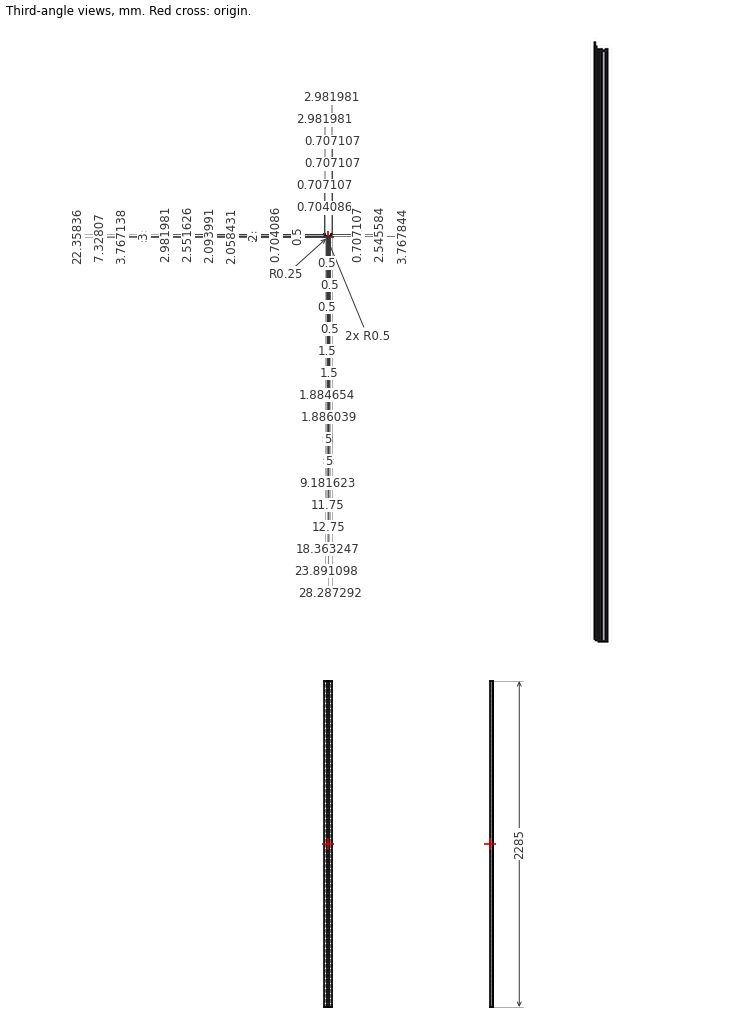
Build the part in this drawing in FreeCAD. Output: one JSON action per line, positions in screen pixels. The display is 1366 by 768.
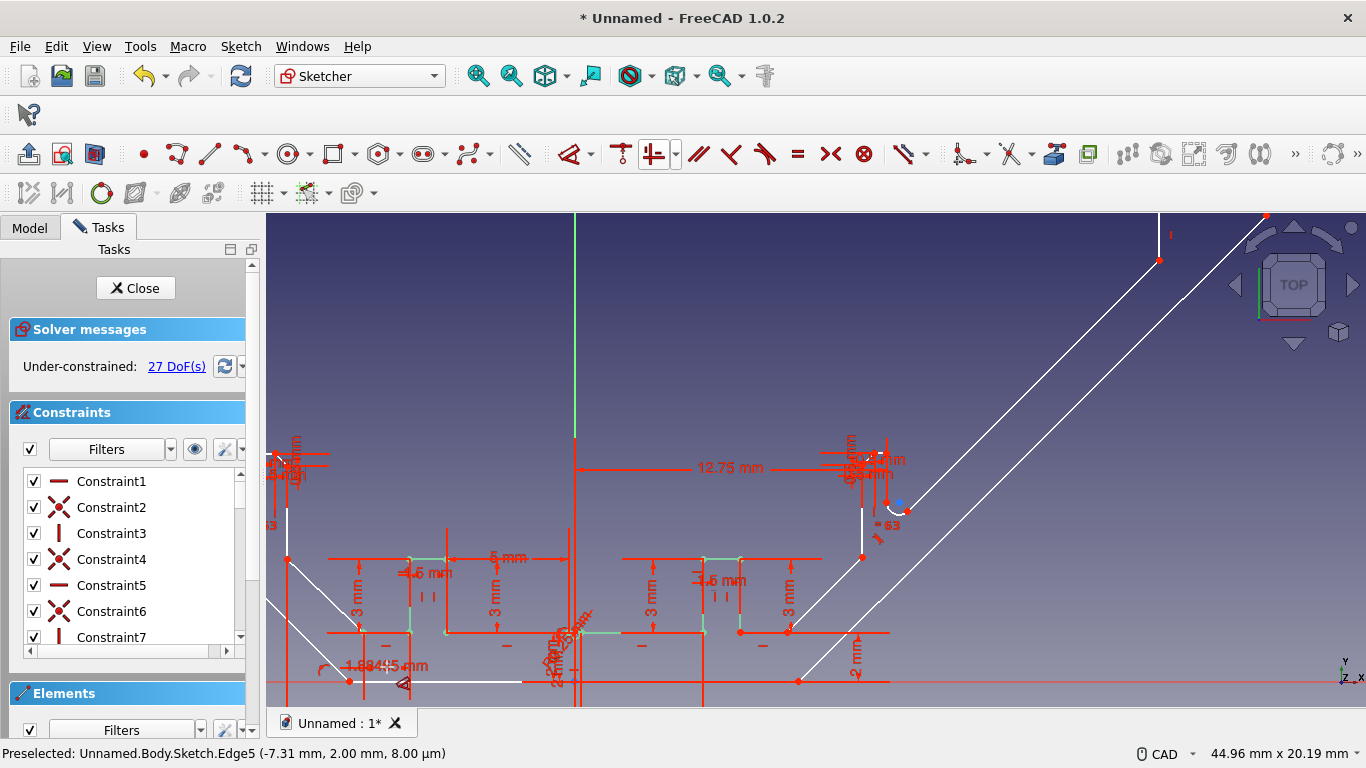
{"action": "scroll", "coordinate": [888, 502], "scroll_direction": "down", "scroll_amount": 4}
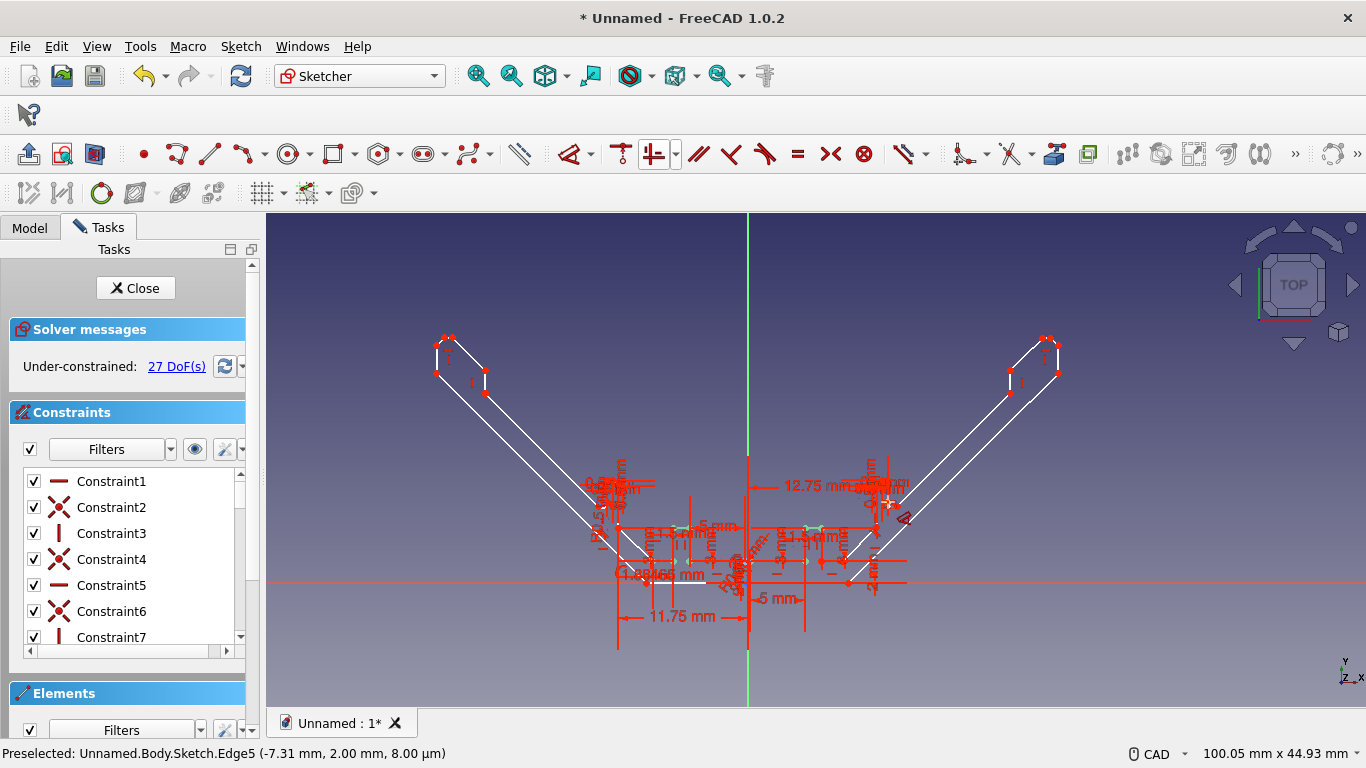
{"action": "left_click", "coordinate": [618, 516]}
{"action": "left_click", "coordinate": [536, 493]}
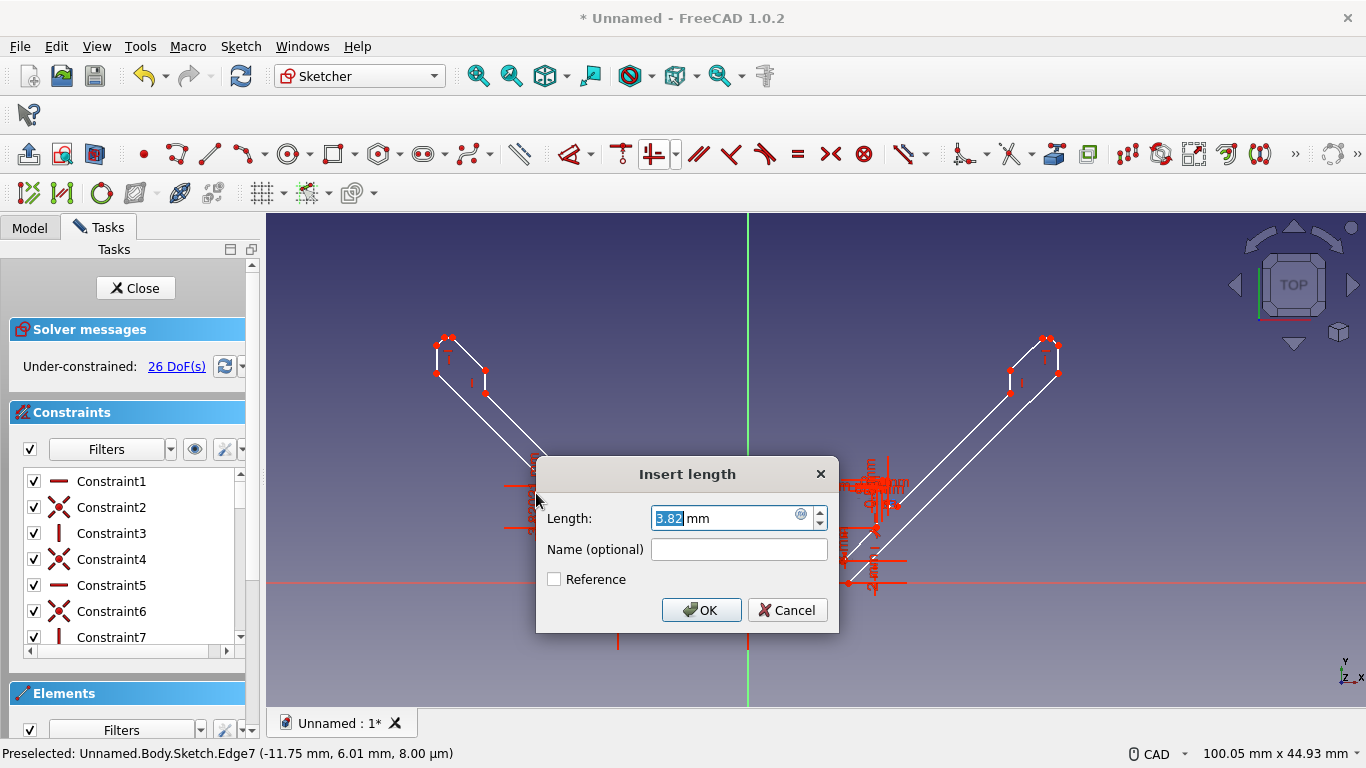
{"action": "type", "text": "3.767138"}
{"action": "key", "text": "Return"}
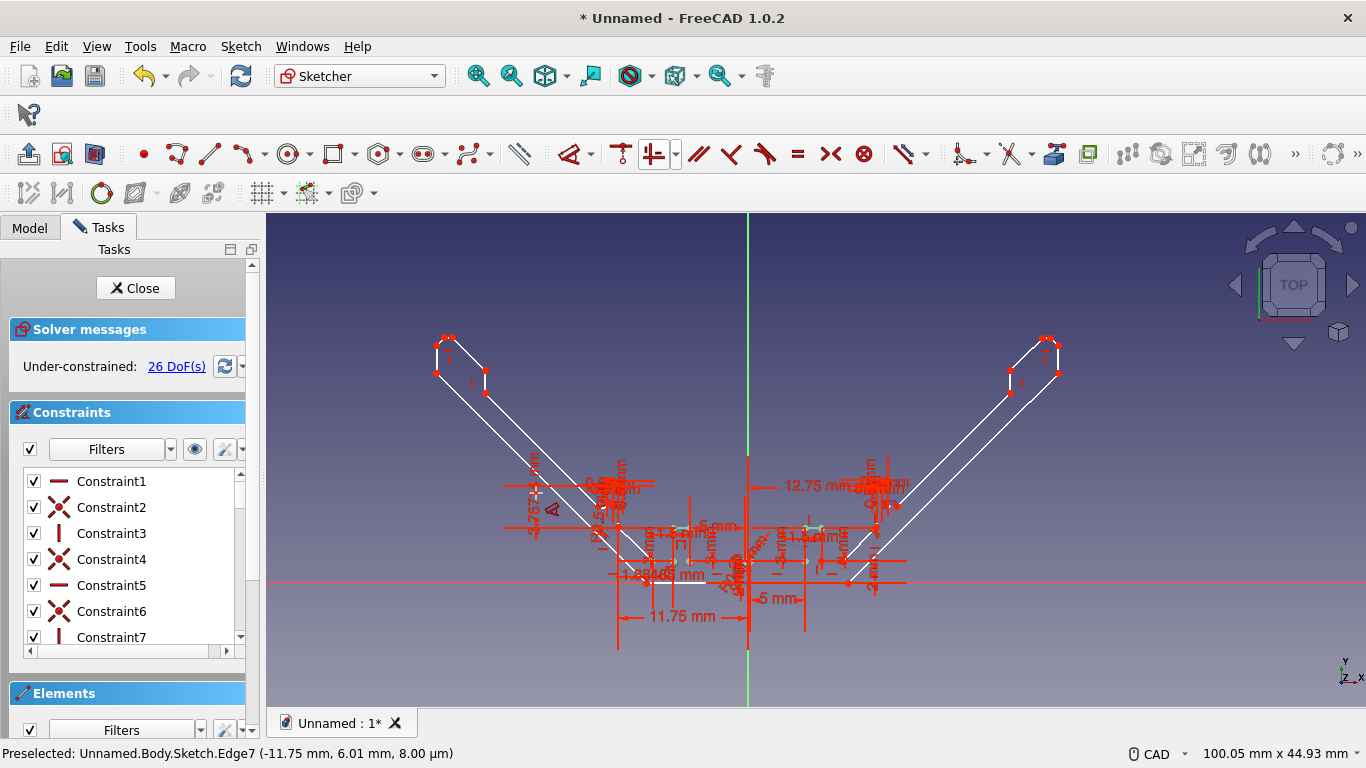
{"action": "scroll", "coordinate": [607, 492], "scroll_direction": "up", "scroll_amount": 3}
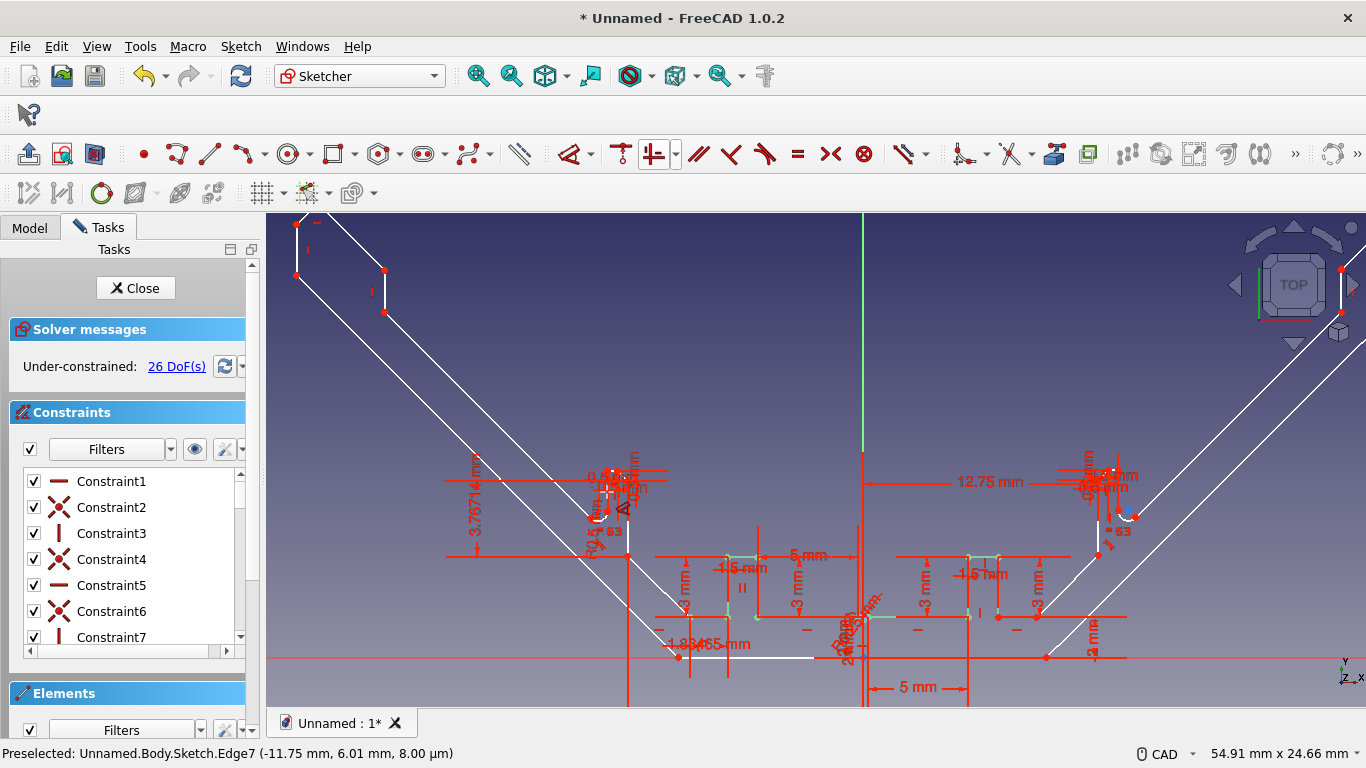
{"action": "left_click", "coordinate": [608, 491]}
{"action": "left_click", "coordinate": [550, 500]}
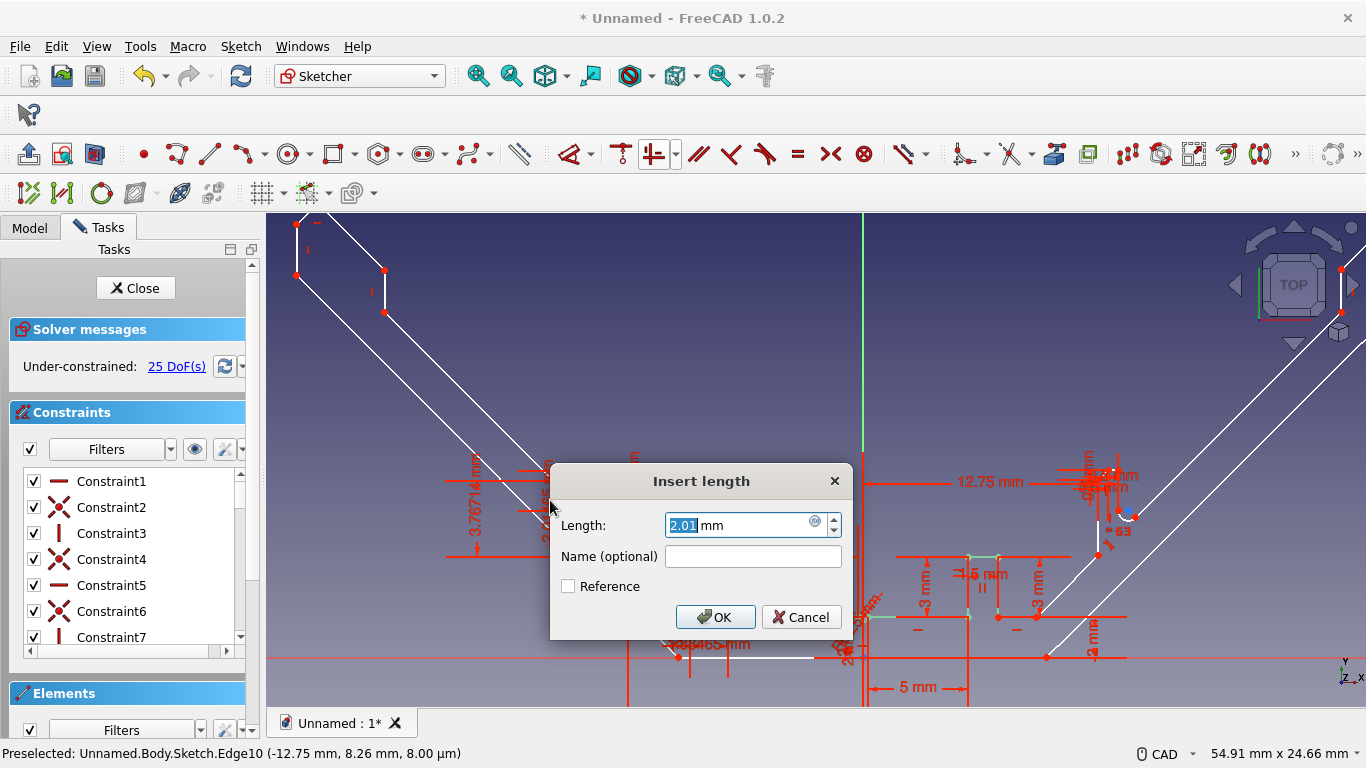
{"action": "type", "text": "2.058431"}
{"action": "key", "text": "Return"}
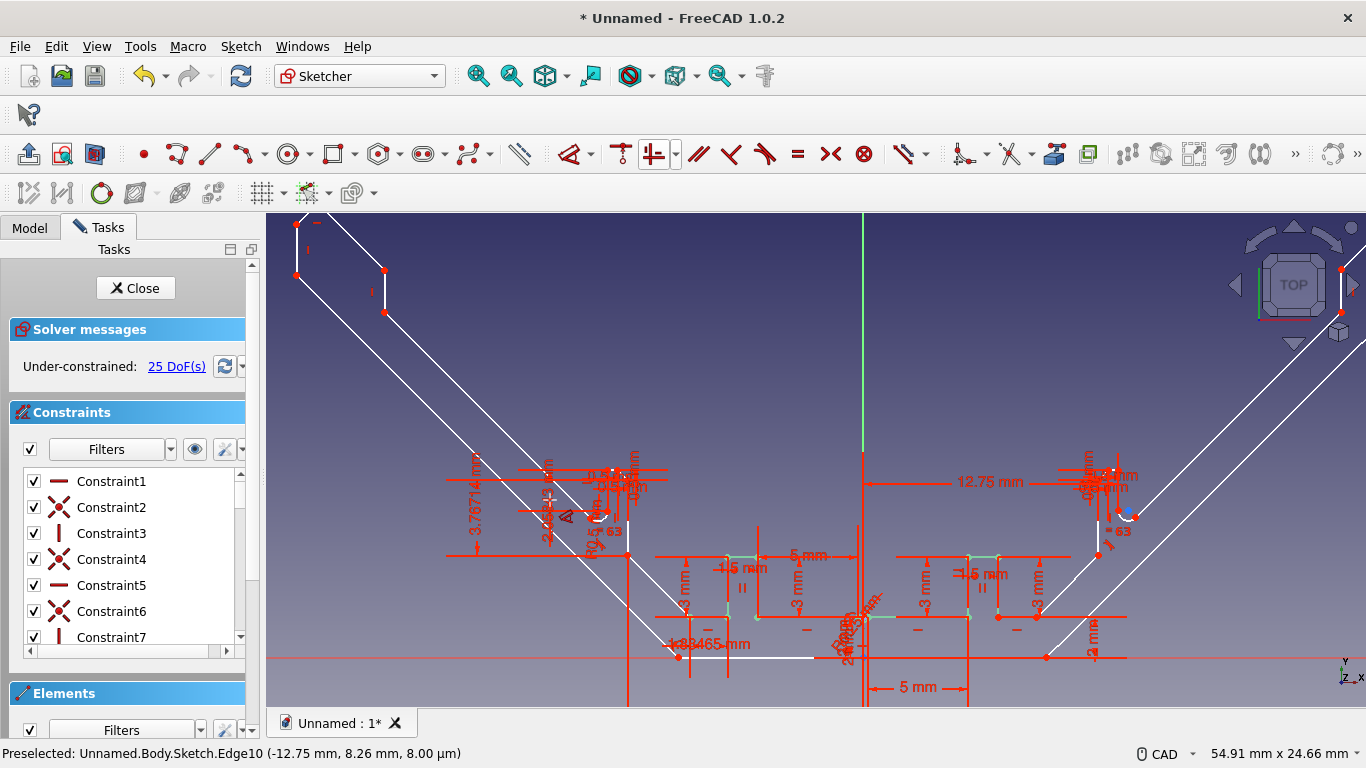
{"action": "left_click", "coordinate": [385, 300]}
{"action": "left_click", "coordinate": [351, 292]}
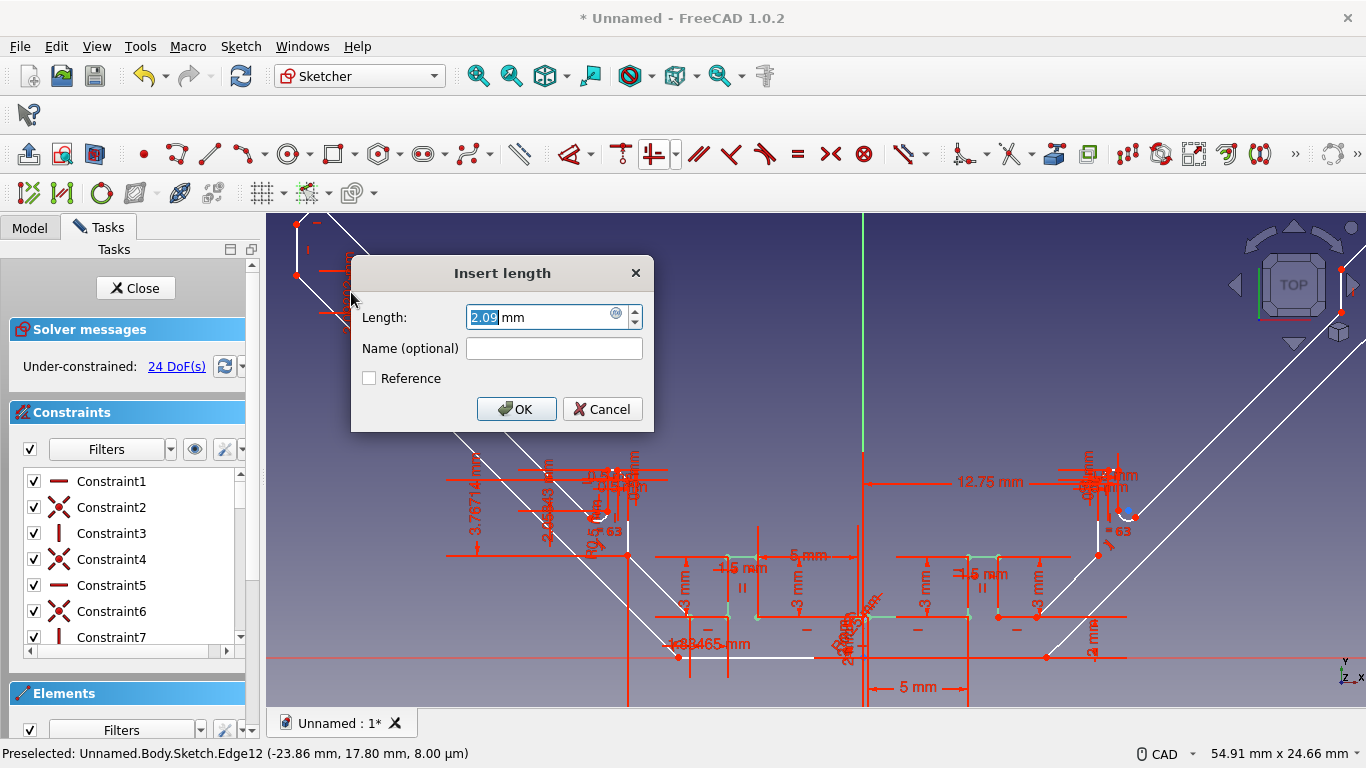
{"action": "type", "text": "2.093991"}
{"action": "key", "text": "Return"}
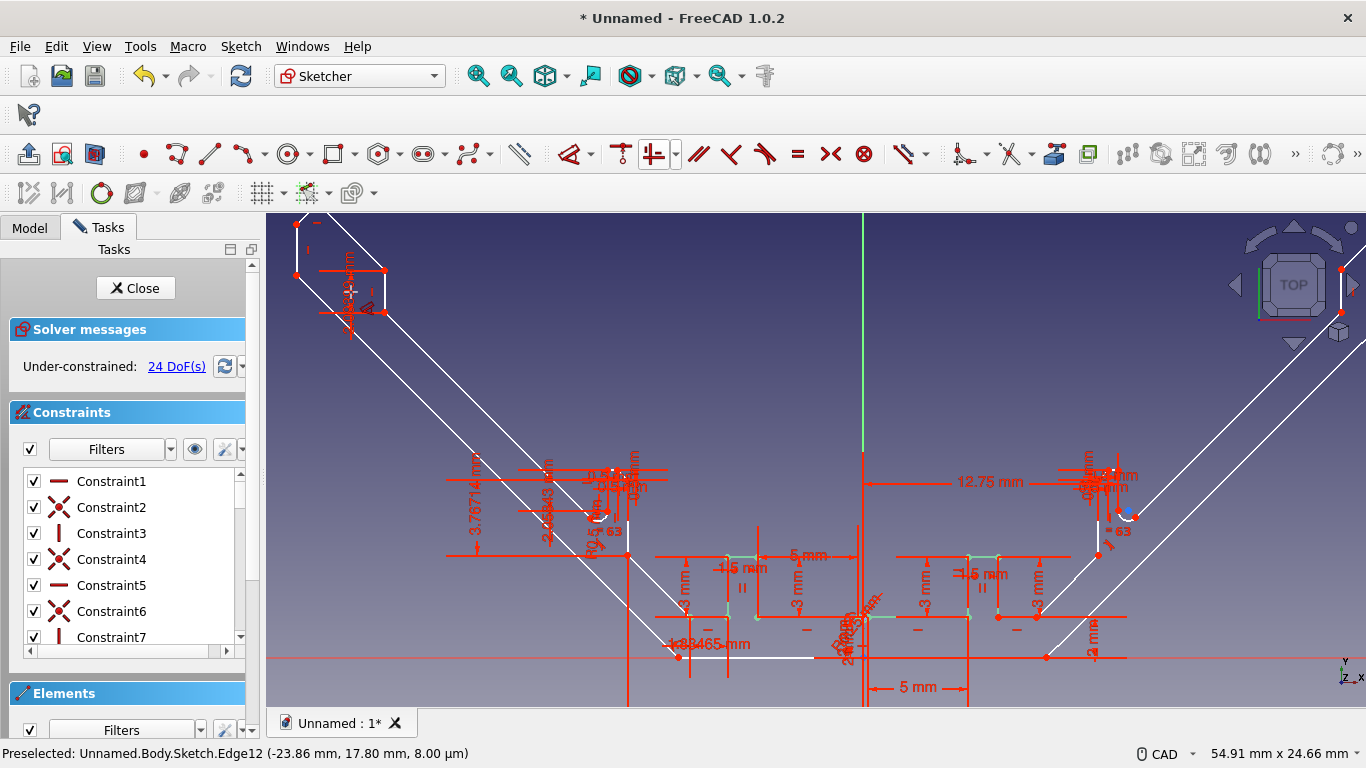
{"action": "scroll", "coordinate": [607, 492], "scroll_direction": "down", "scroll_amount": 3}